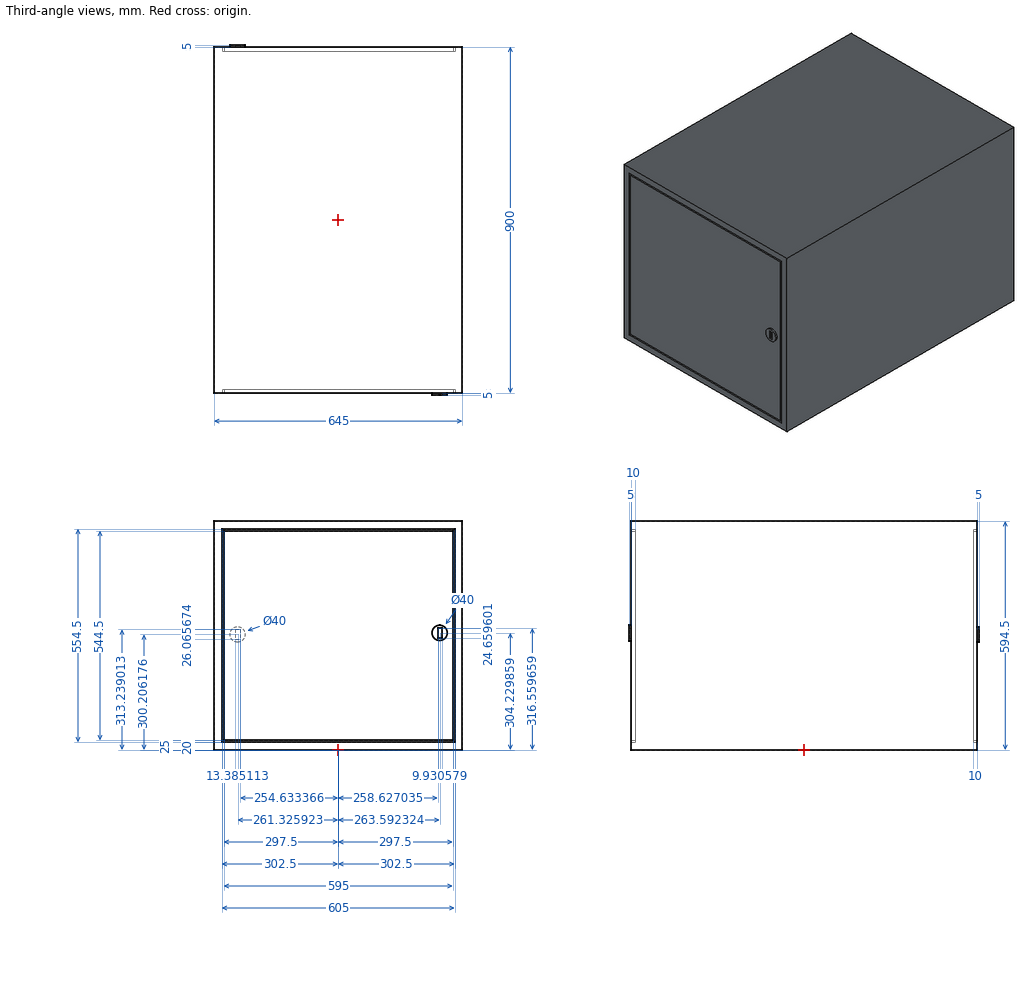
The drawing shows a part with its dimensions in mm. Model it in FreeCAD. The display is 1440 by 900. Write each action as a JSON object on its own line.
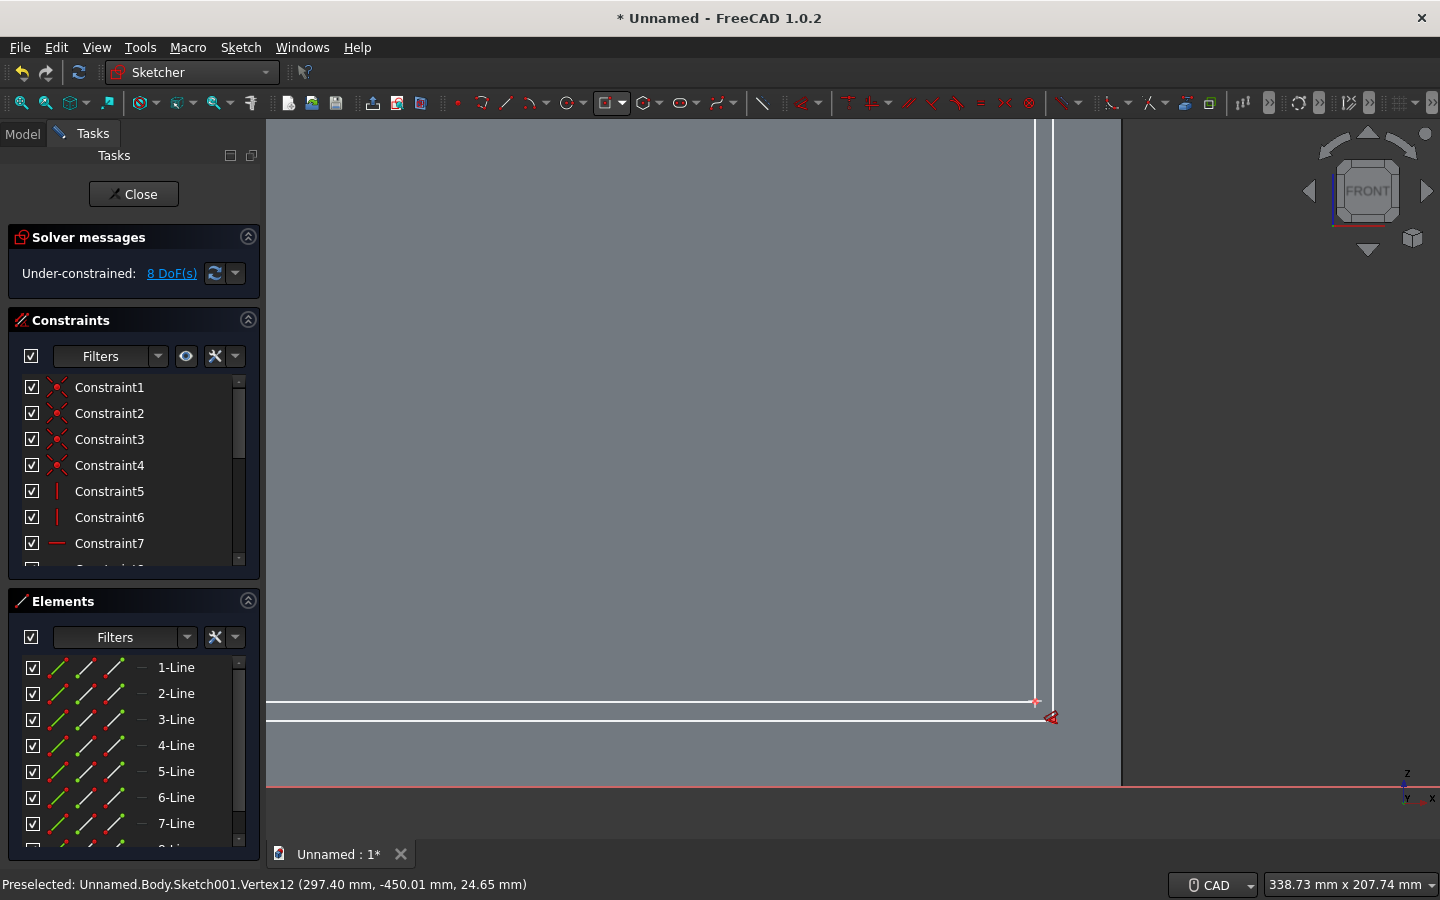
{"action": "left_click", "coordinate": [424, 721]}
{"action": "left_click", "coordinate": [674, 755]}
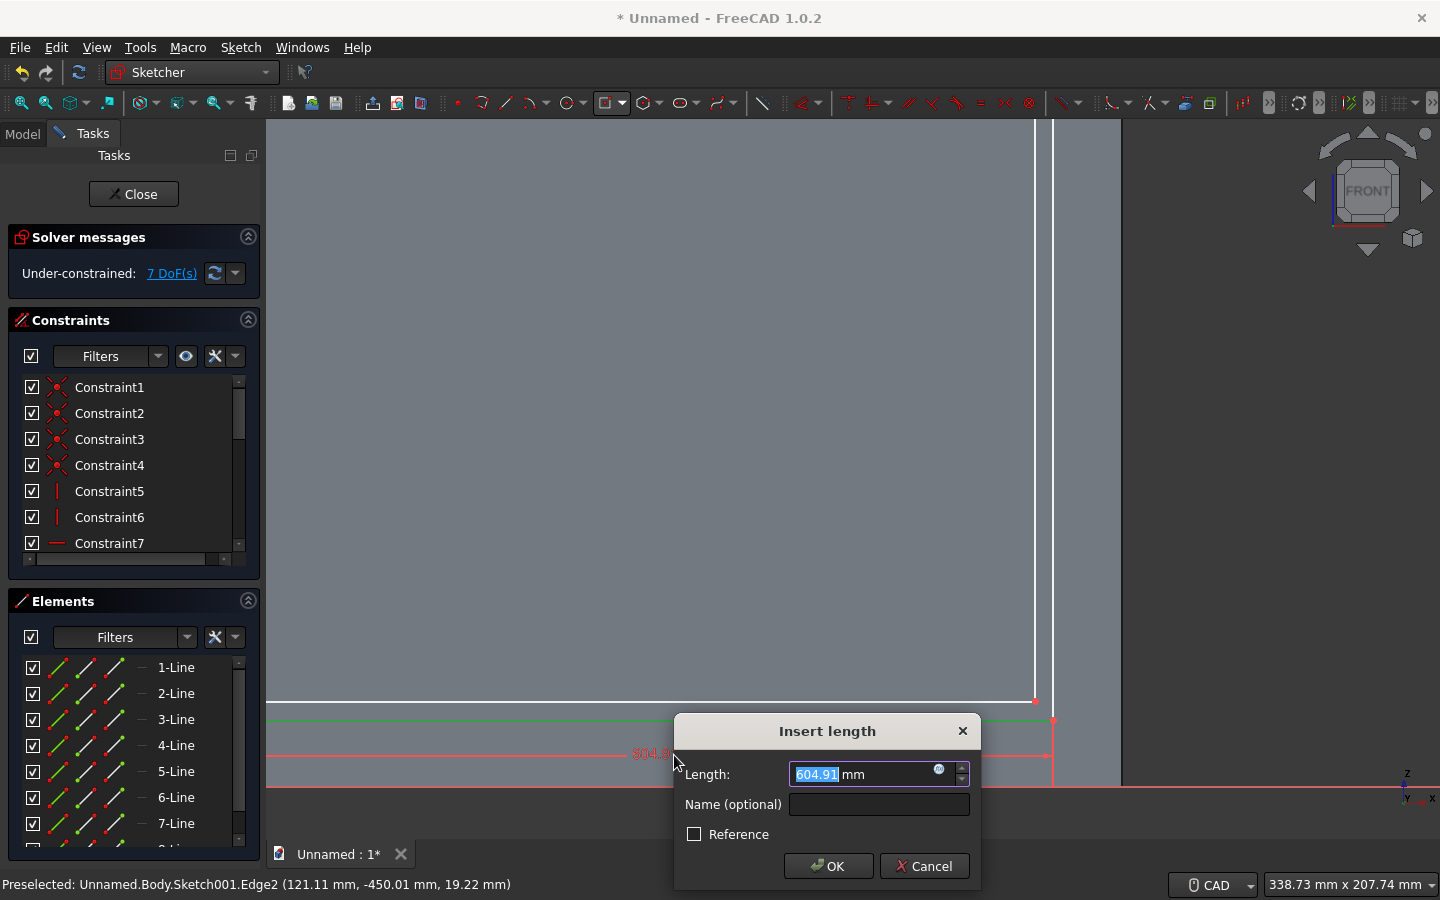
{"action": "type", "text": "605"}
{"action": "key", "text": "Return"}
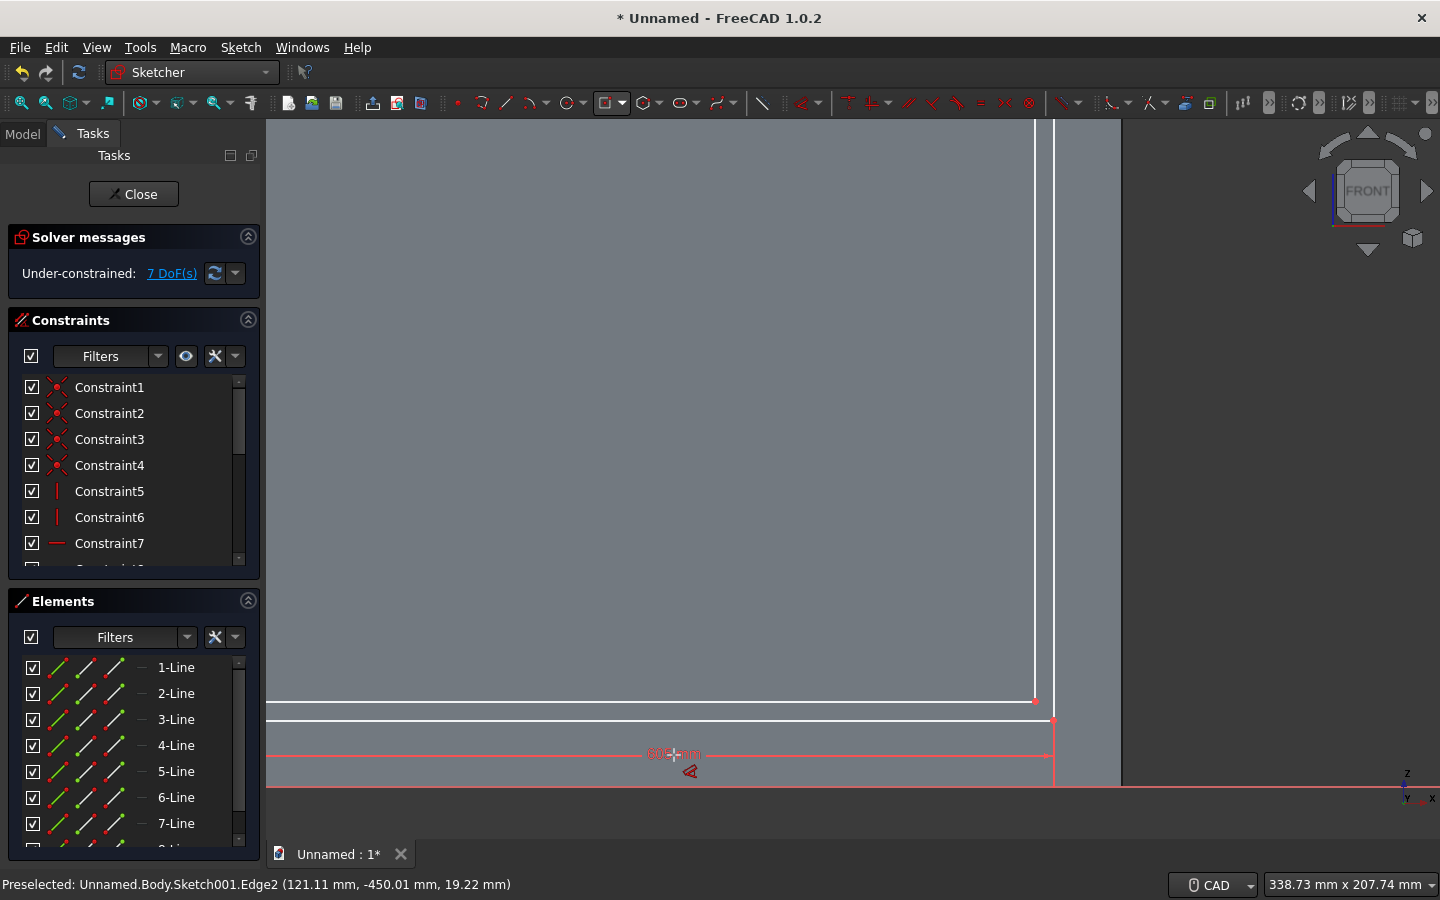
{"action": "left_click", "coordinate": [417, 702]}
{"action": "left_click", "coordinate": [494, 736]}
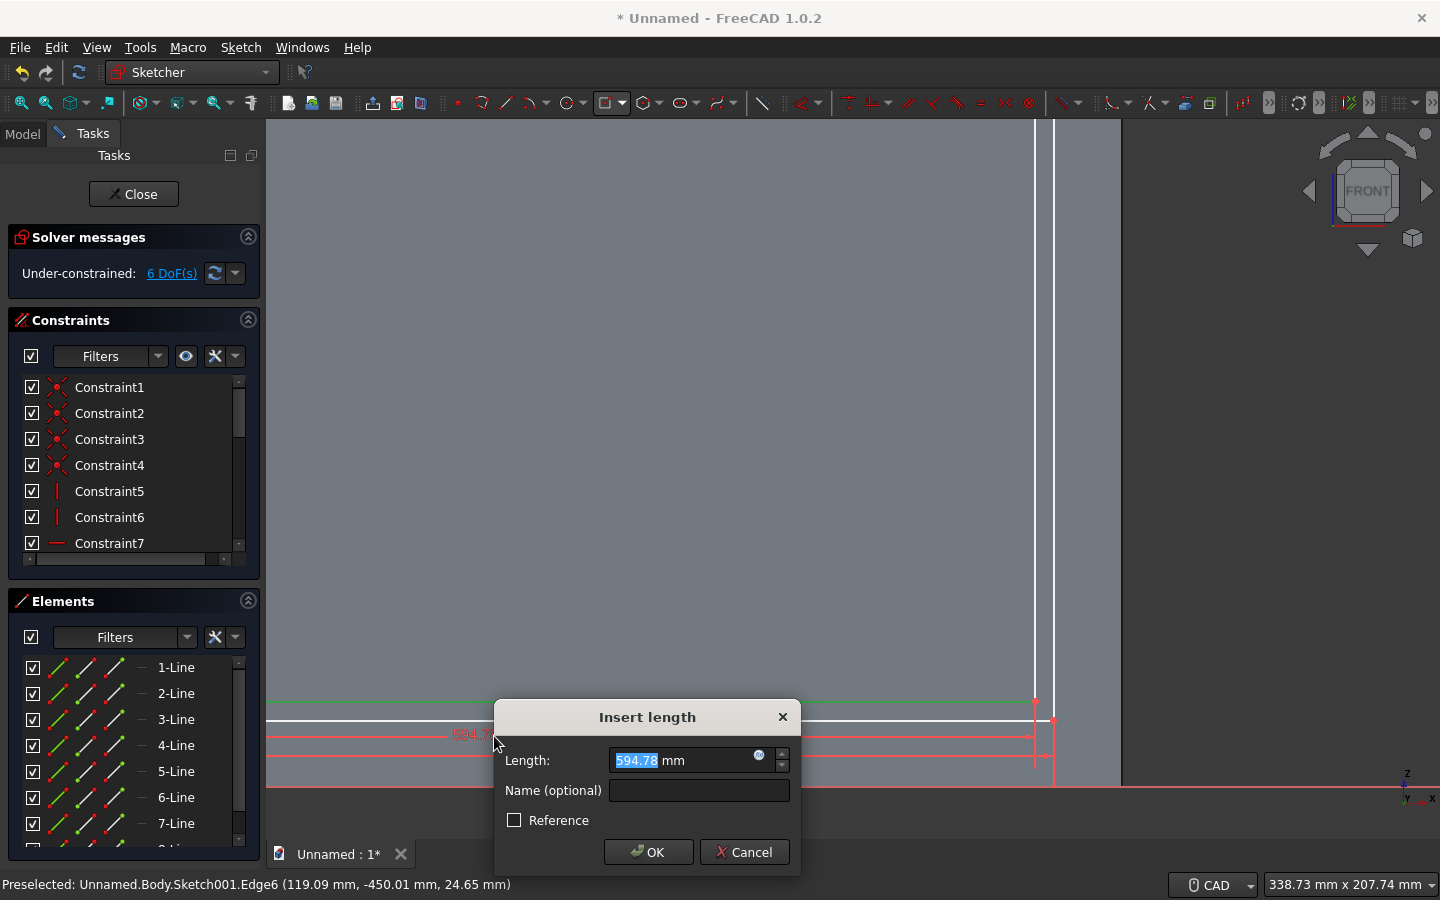
{"action": "type", "text": "595"}
{"action": "key", "text": "Return"}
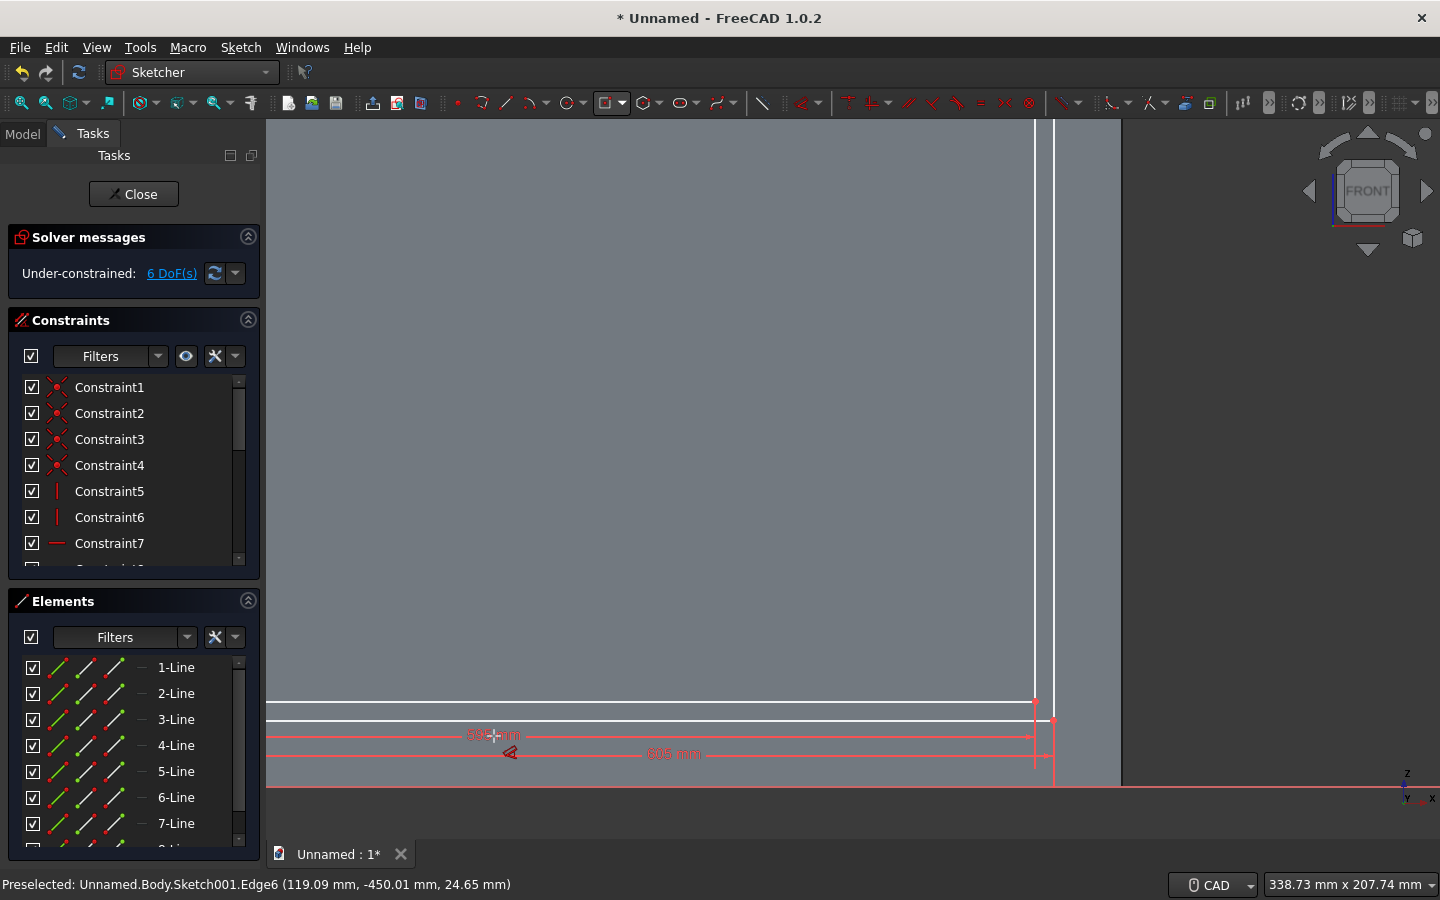
{"action": "scroll", "coordinate": [1040, 704], "scroll_direction": "down", "scroll_amount": 7}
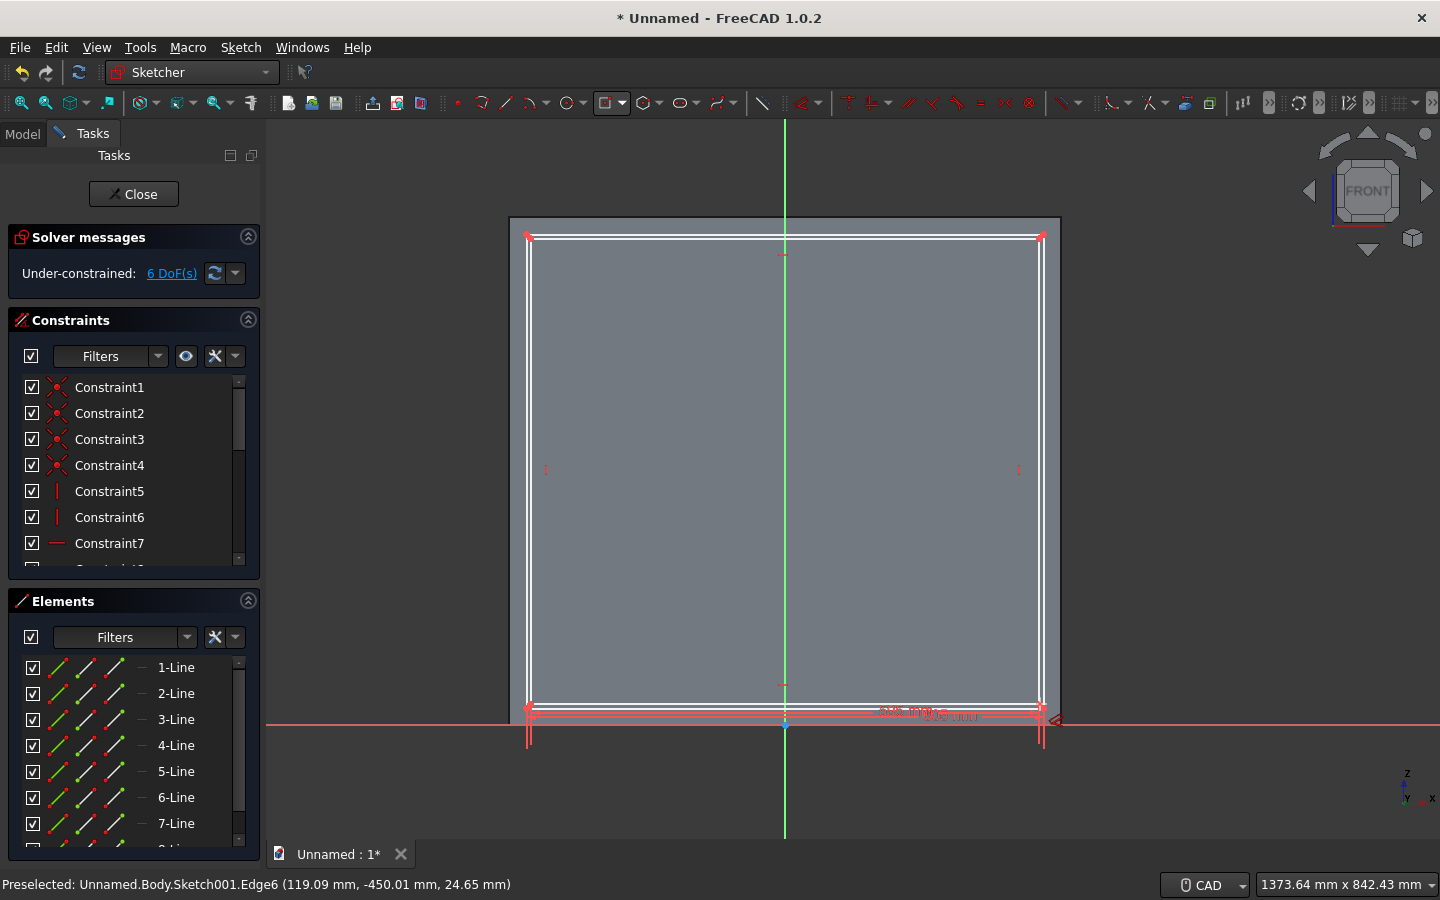
{"action": "scroll", "coordinate": [527, 709], "scroll_direction": "up", "scroll_amount": 5}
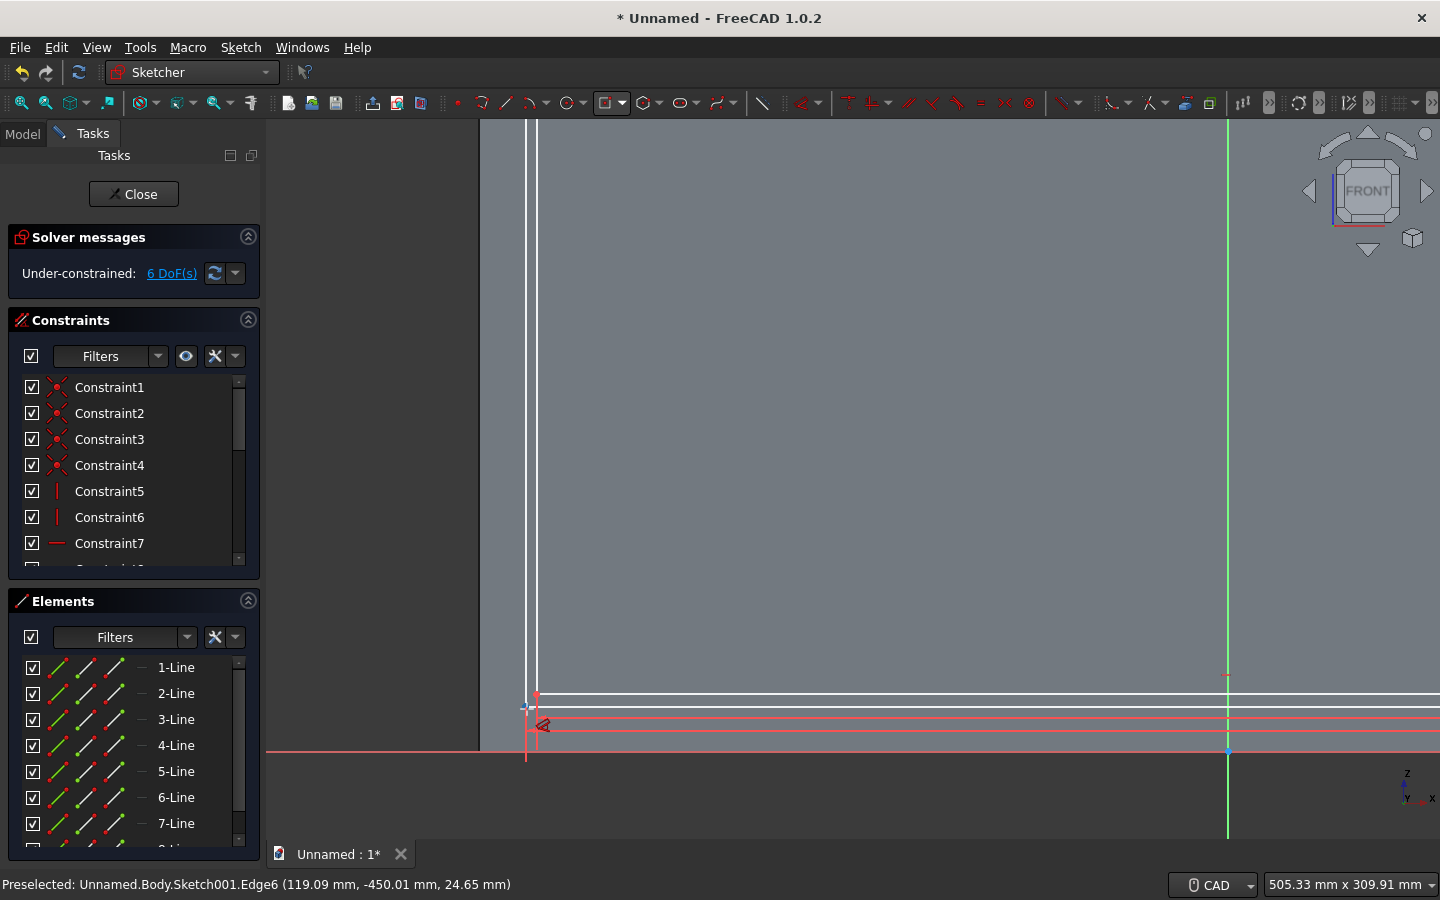
{"action": "left_click", "coordinate": [526, 707]}
{"action": "left_click", "coordinate": [492, 729]}